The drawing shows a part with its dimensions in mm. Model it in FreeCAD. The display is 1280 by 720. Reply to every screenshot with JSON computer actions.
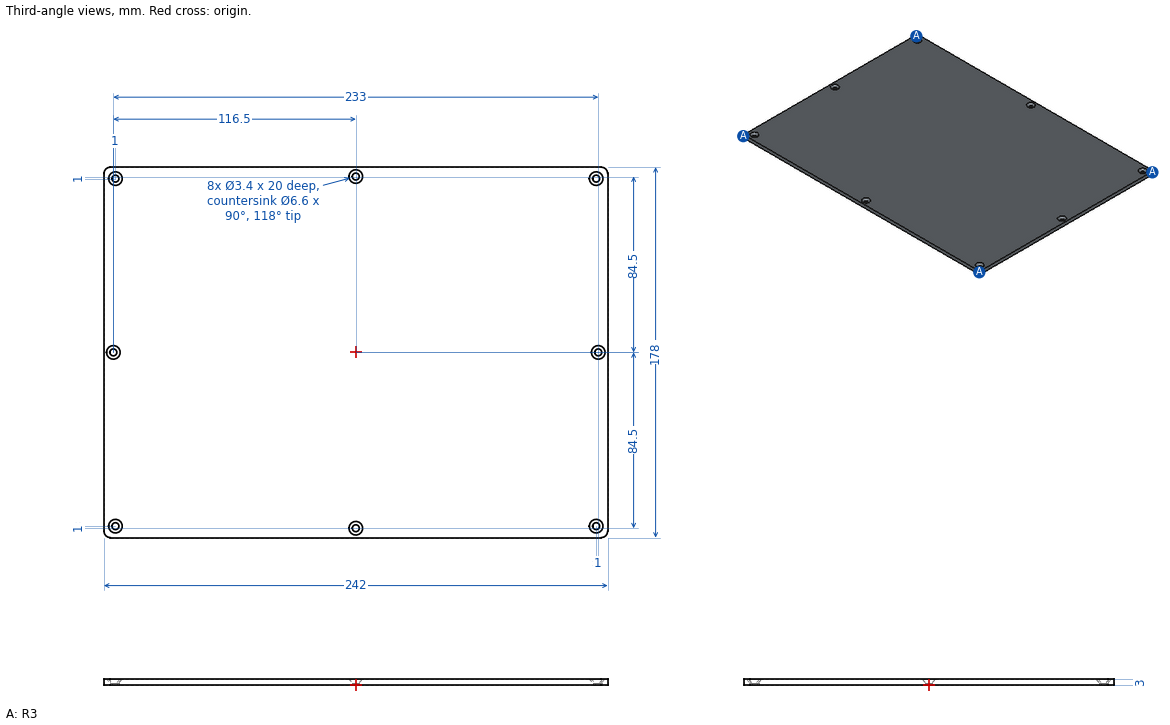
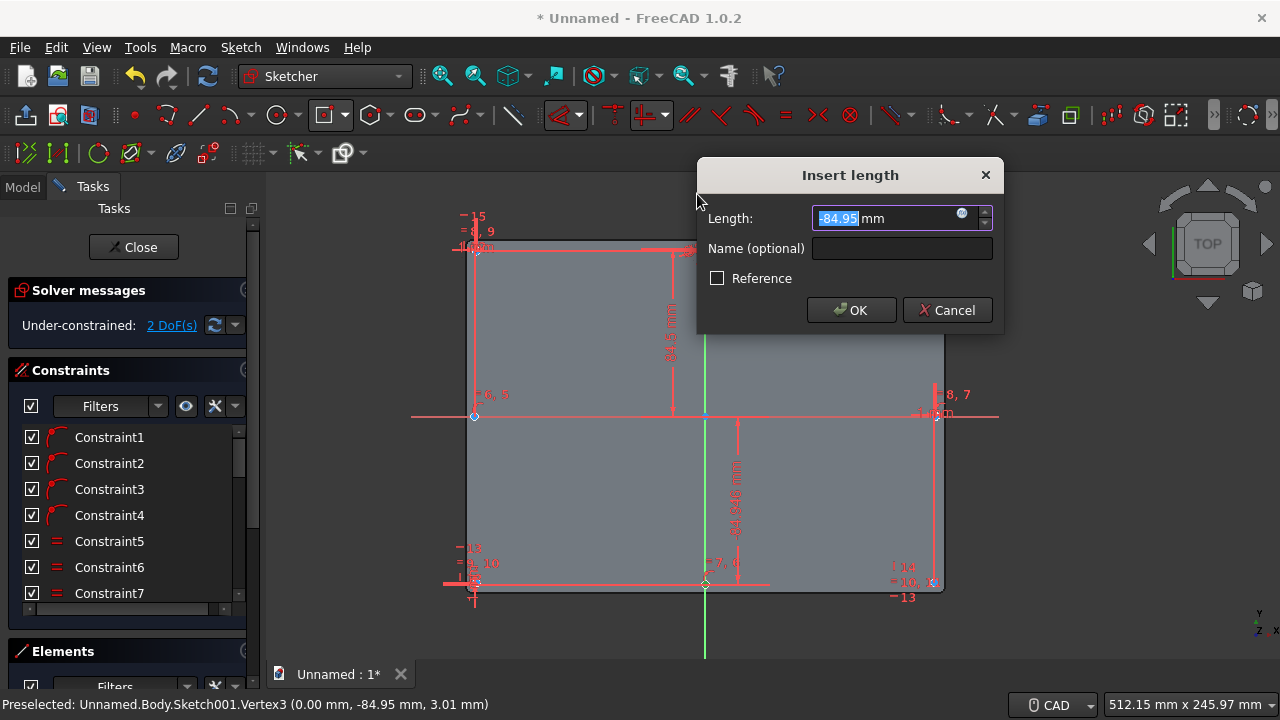
{"action": "type", "text": "-84.5"}
{"action": "key", "text": "Return"}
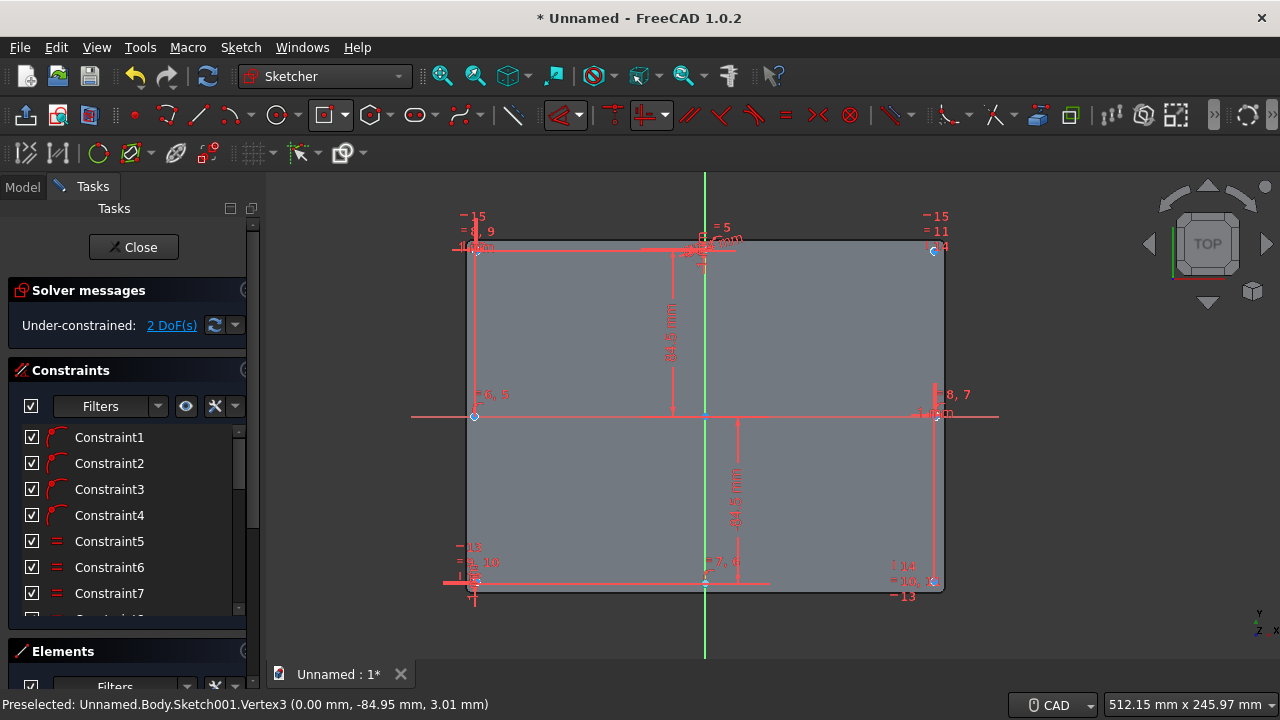
{"action": "left_click", "coordinate": [475, 417]}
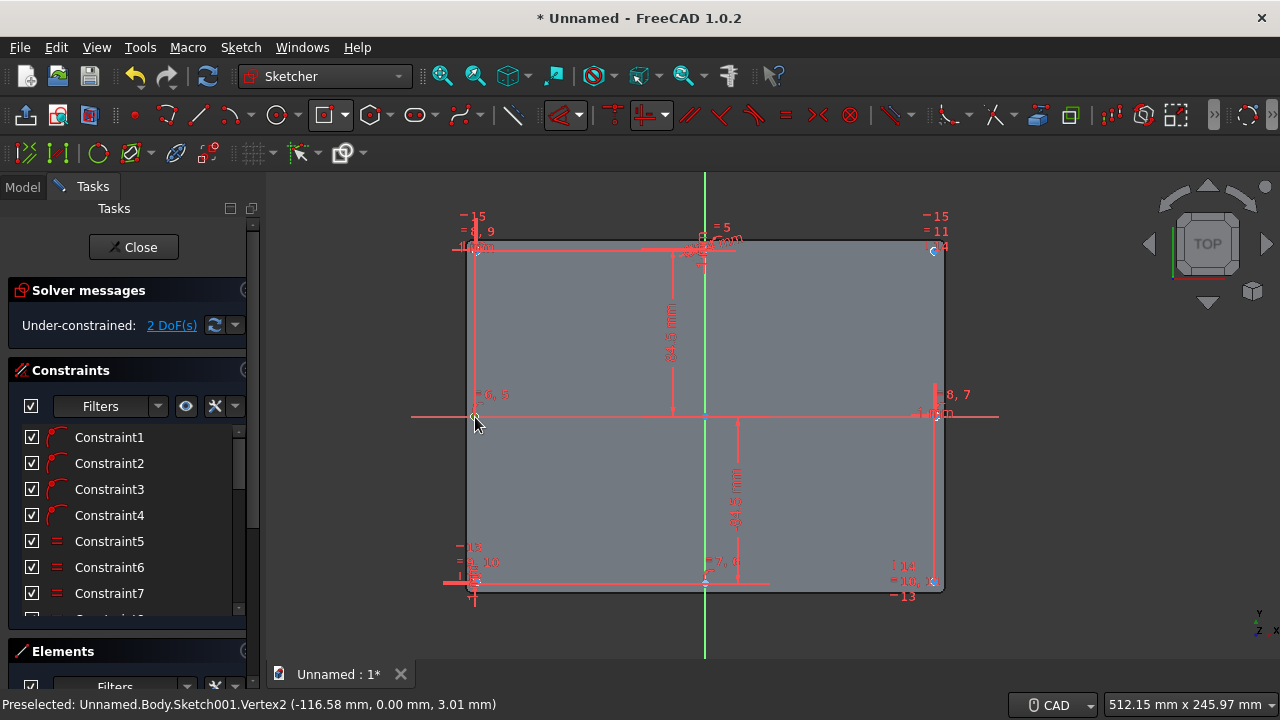
{"action": "left_click", "coordinate": [936, 417]}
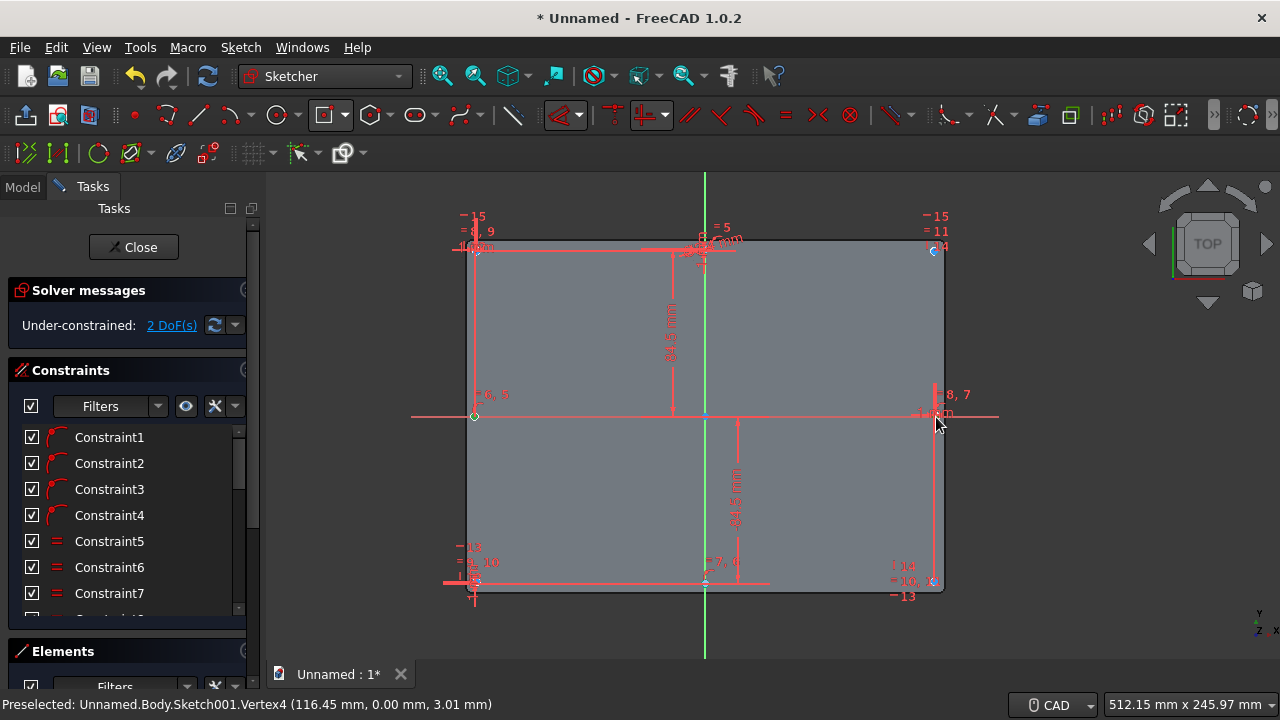
{"action": "key", "text": "l"}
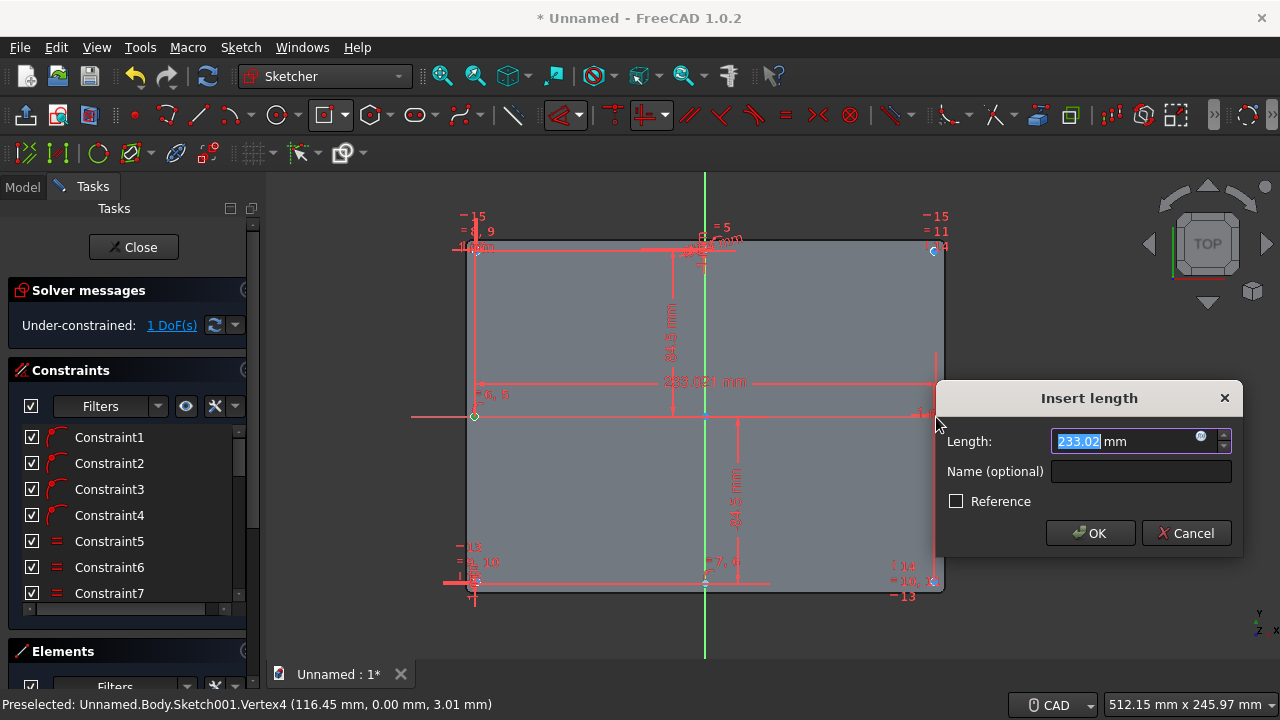
{"action": "type", "text": "233"}
{"action": "key", "text": "Return"}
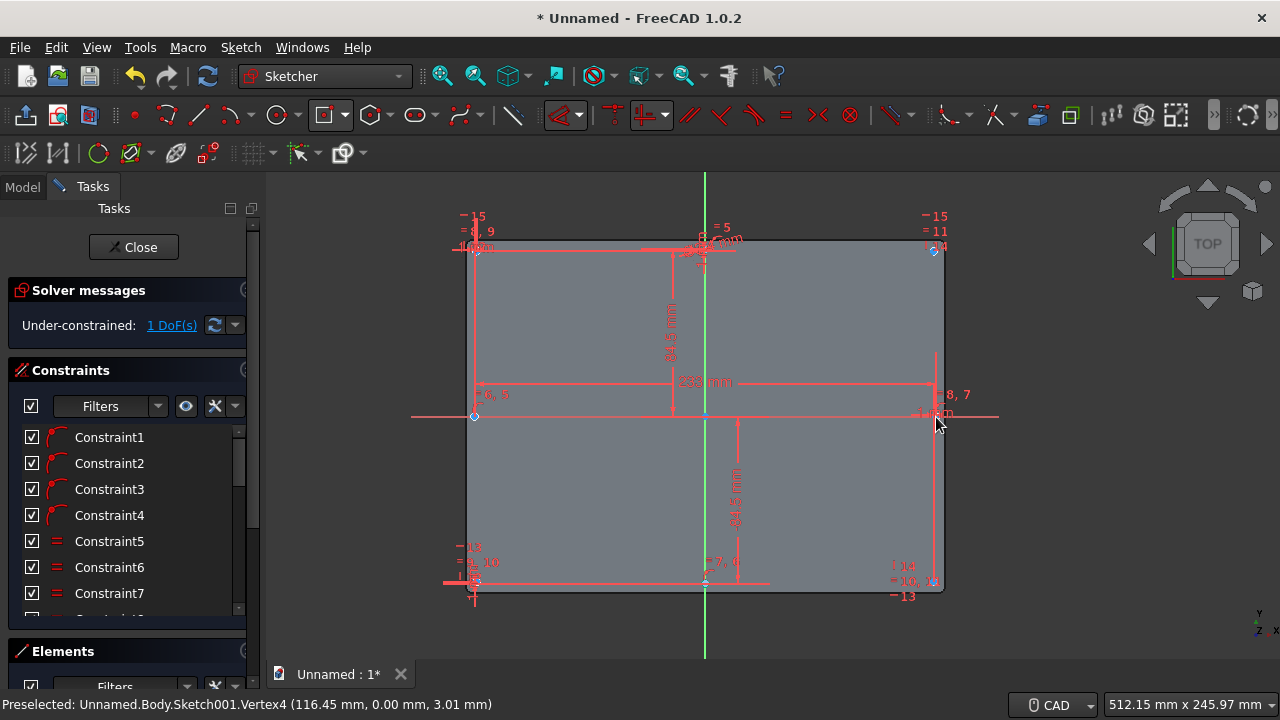
{"action": "left_click", "coordinate": [475, 417]}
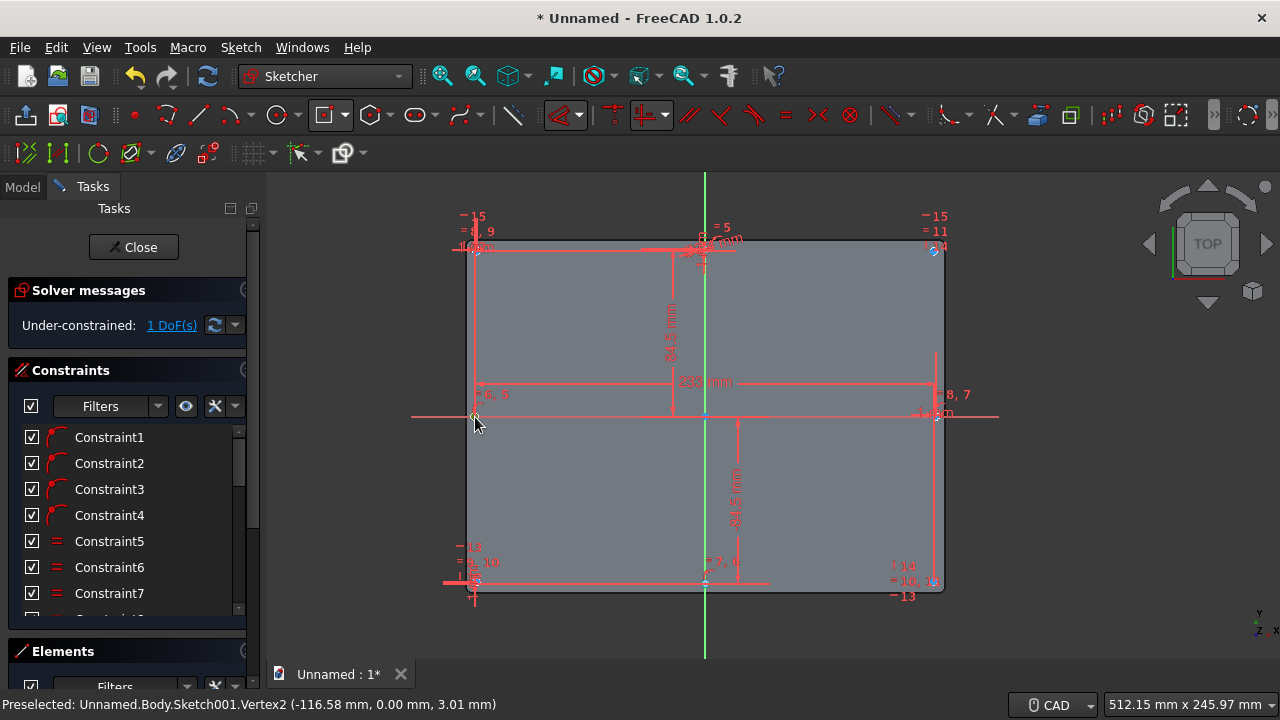
{"action": "left_click", "coordinate": [582, 116]}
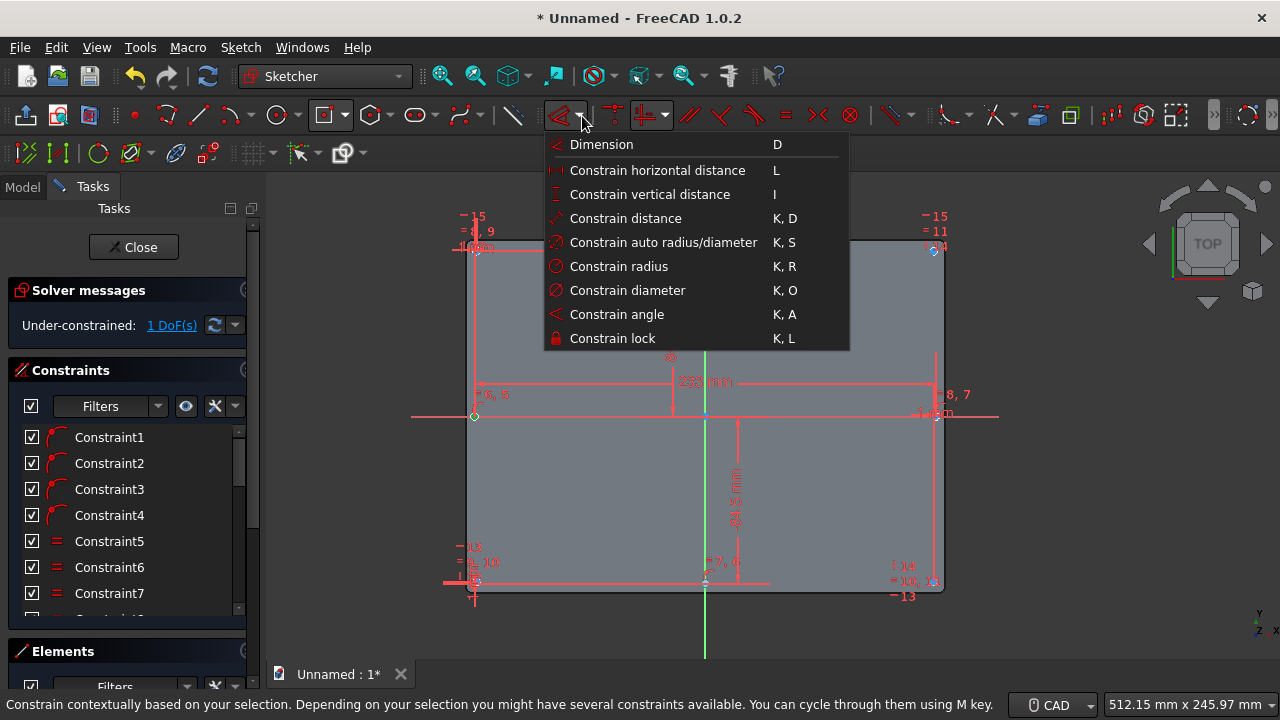
{"action": "left_click", "coordinate": [697, 170]}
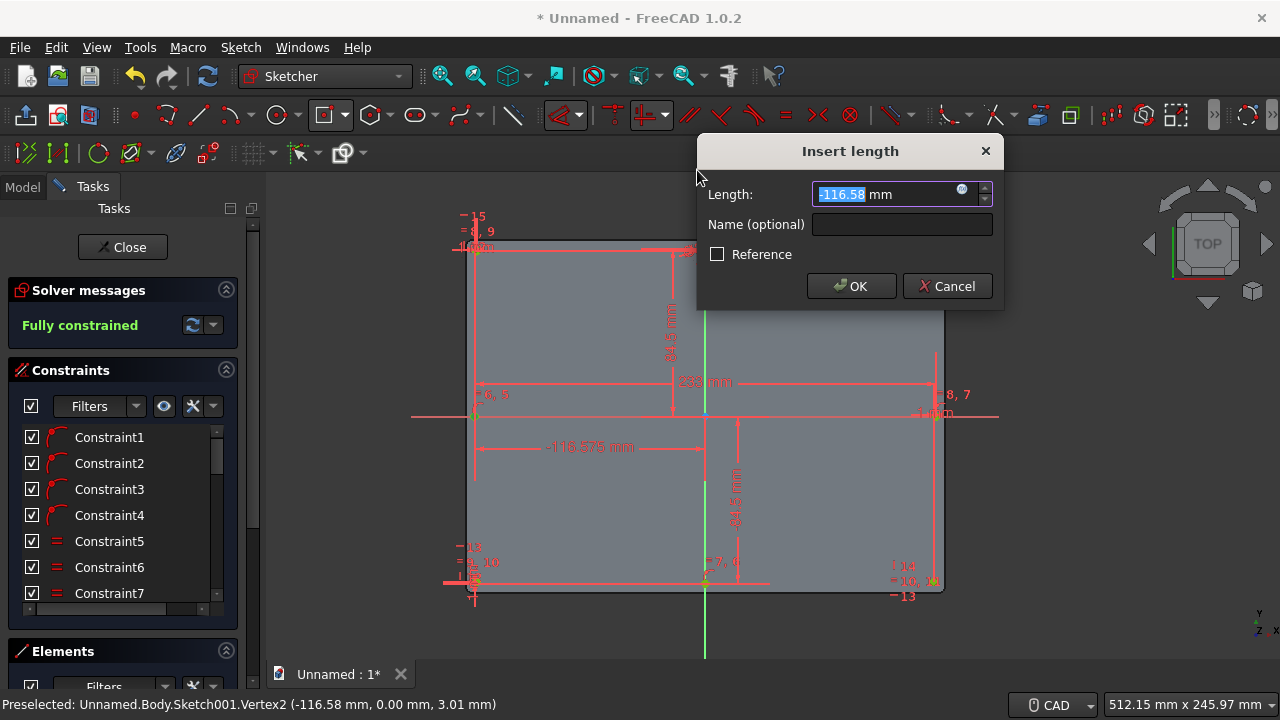
{"action": "type", "text": "-116.5"}
{"action": "key", "text": "Return"}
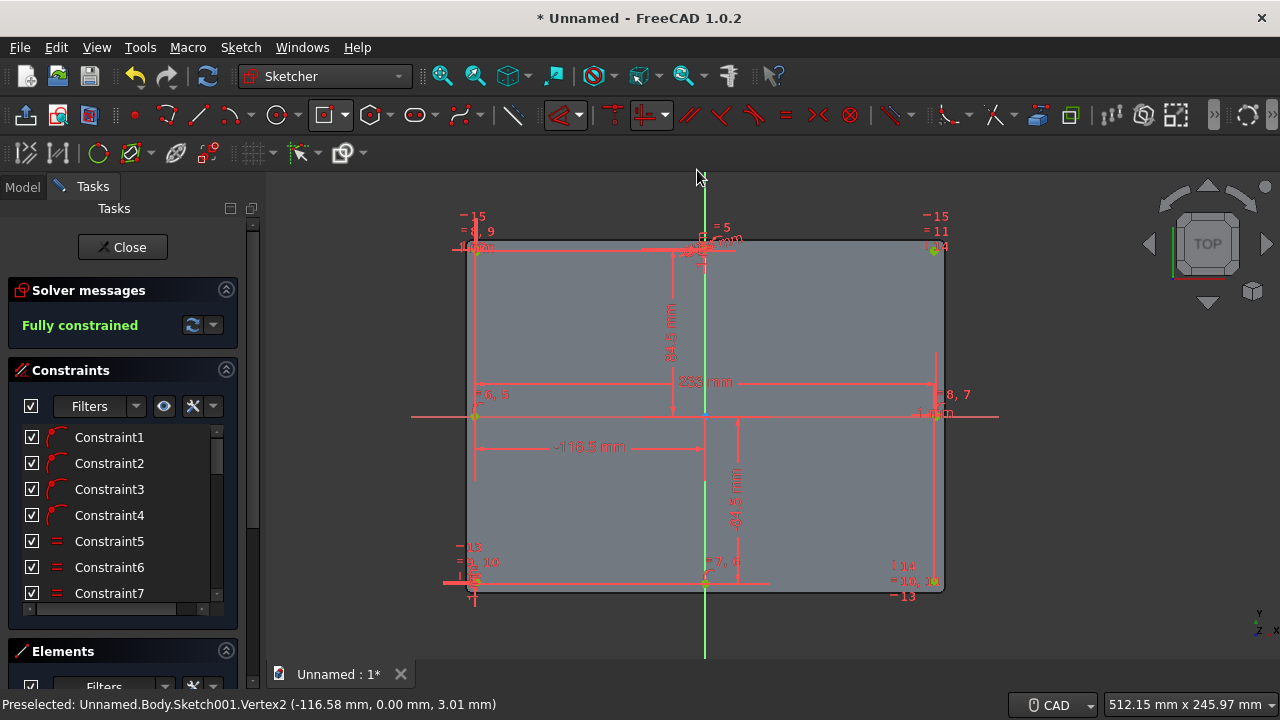
{"action": "left_click", "coordinate": [123, 247]}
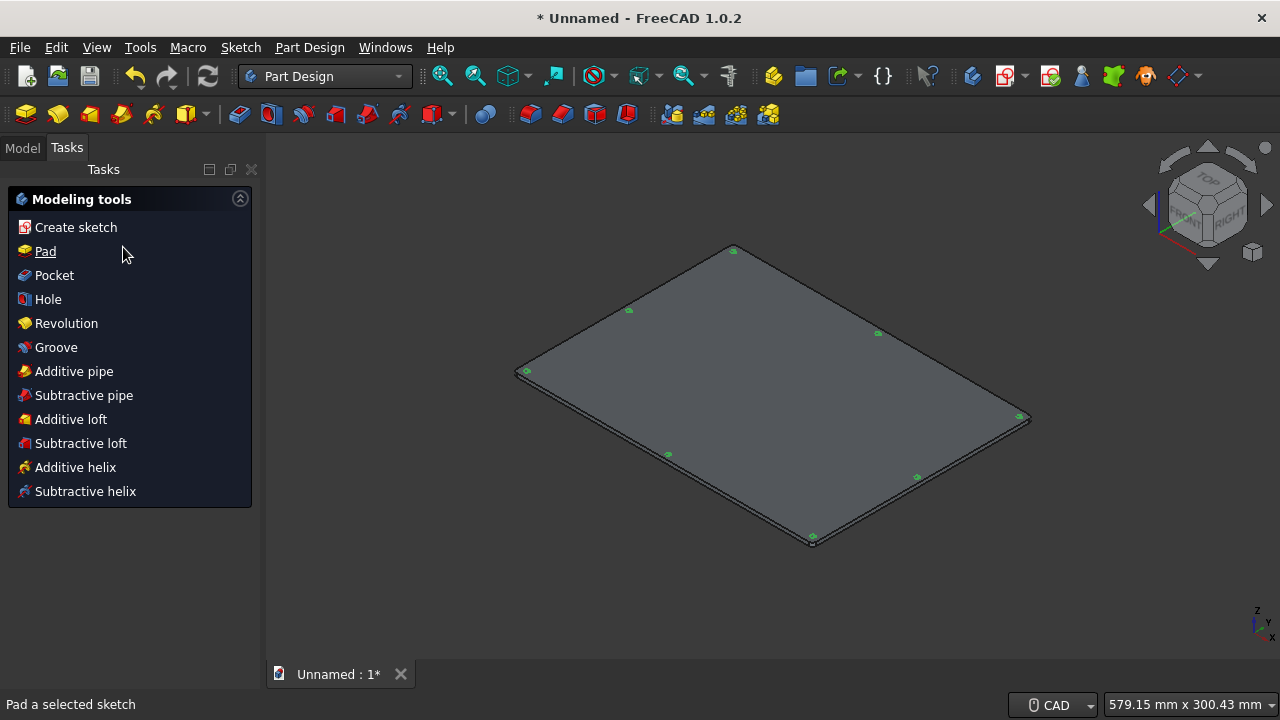
{"action": "left_click", "coordinate": [272, 114]}